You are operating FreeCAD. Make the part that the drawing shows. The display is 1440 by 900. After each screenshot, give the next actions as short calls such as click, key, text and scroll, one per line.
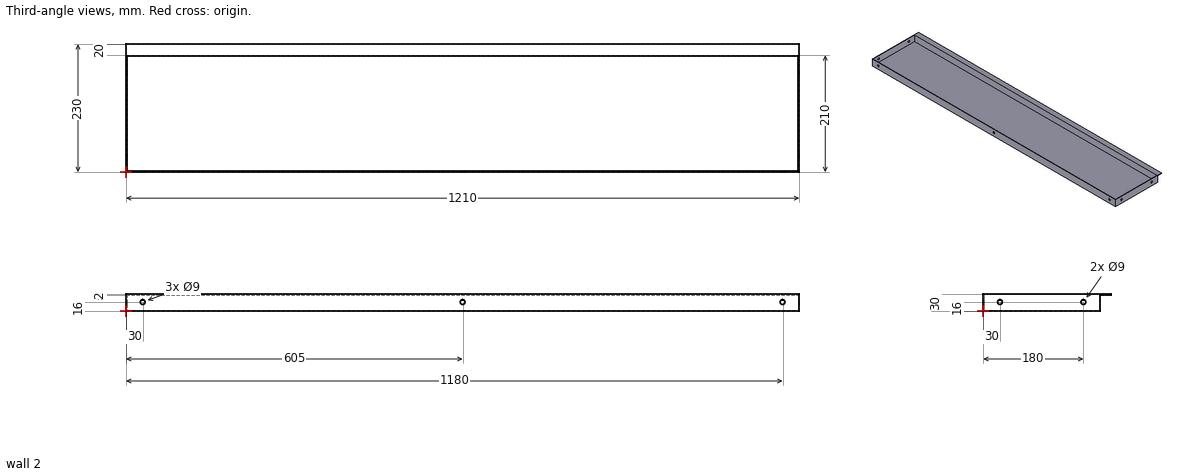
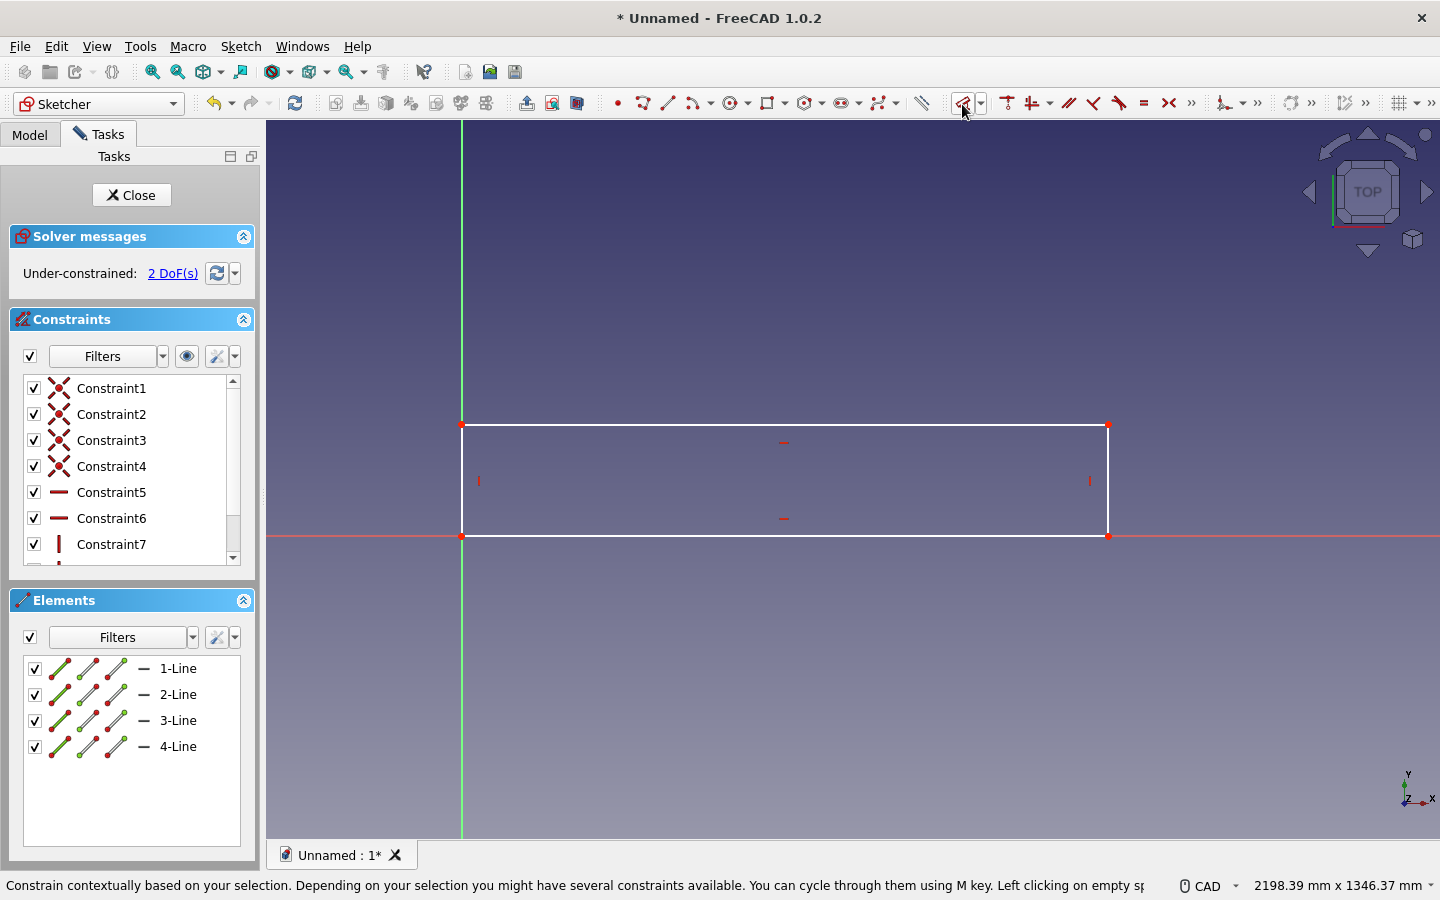
click(1108, 503)
click(1142, 481)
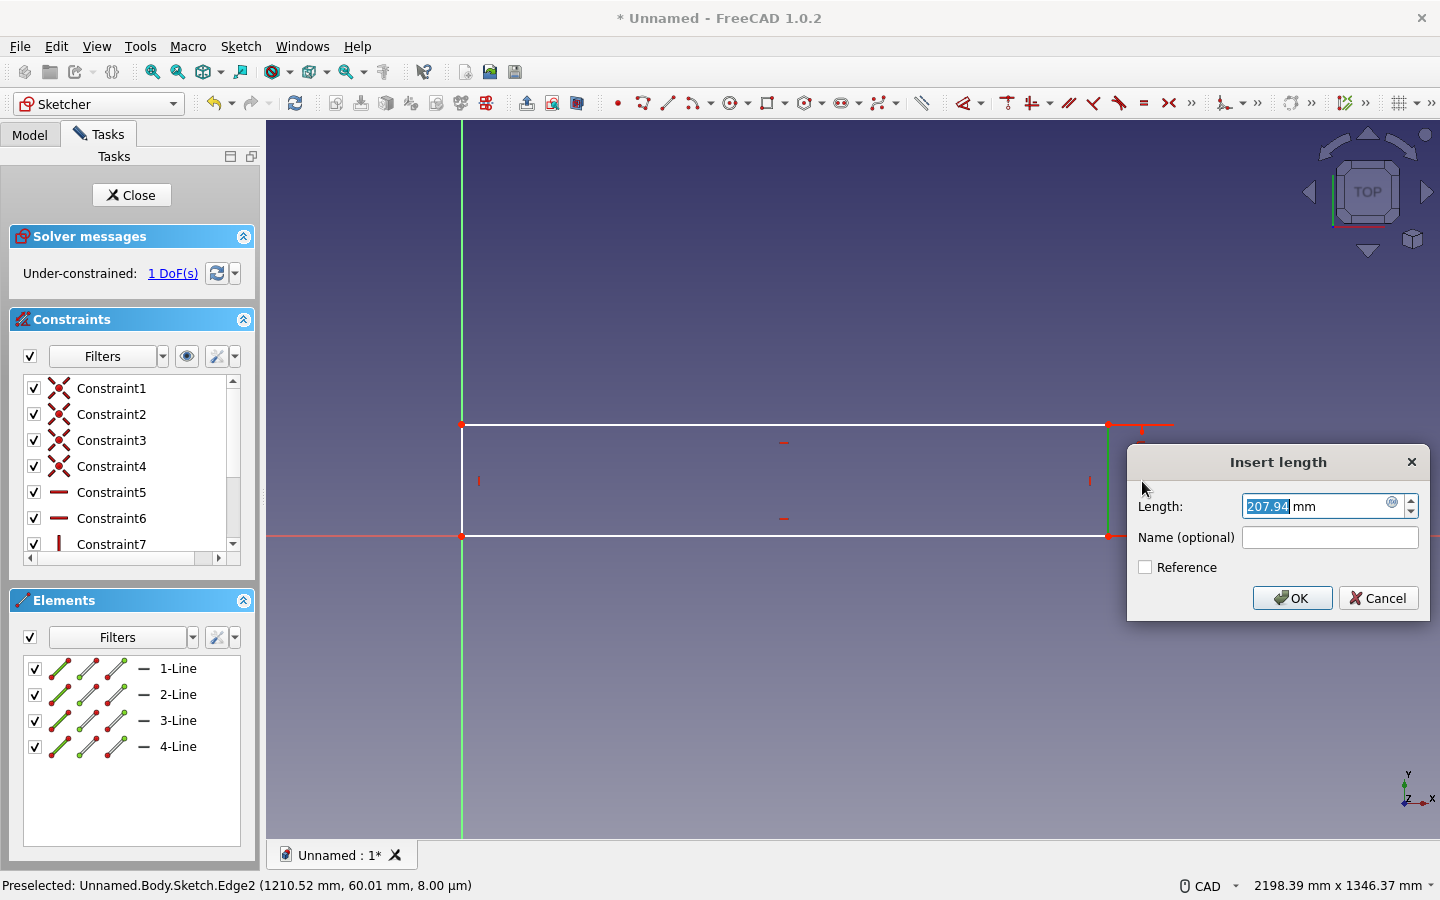
text(210)
key(Return)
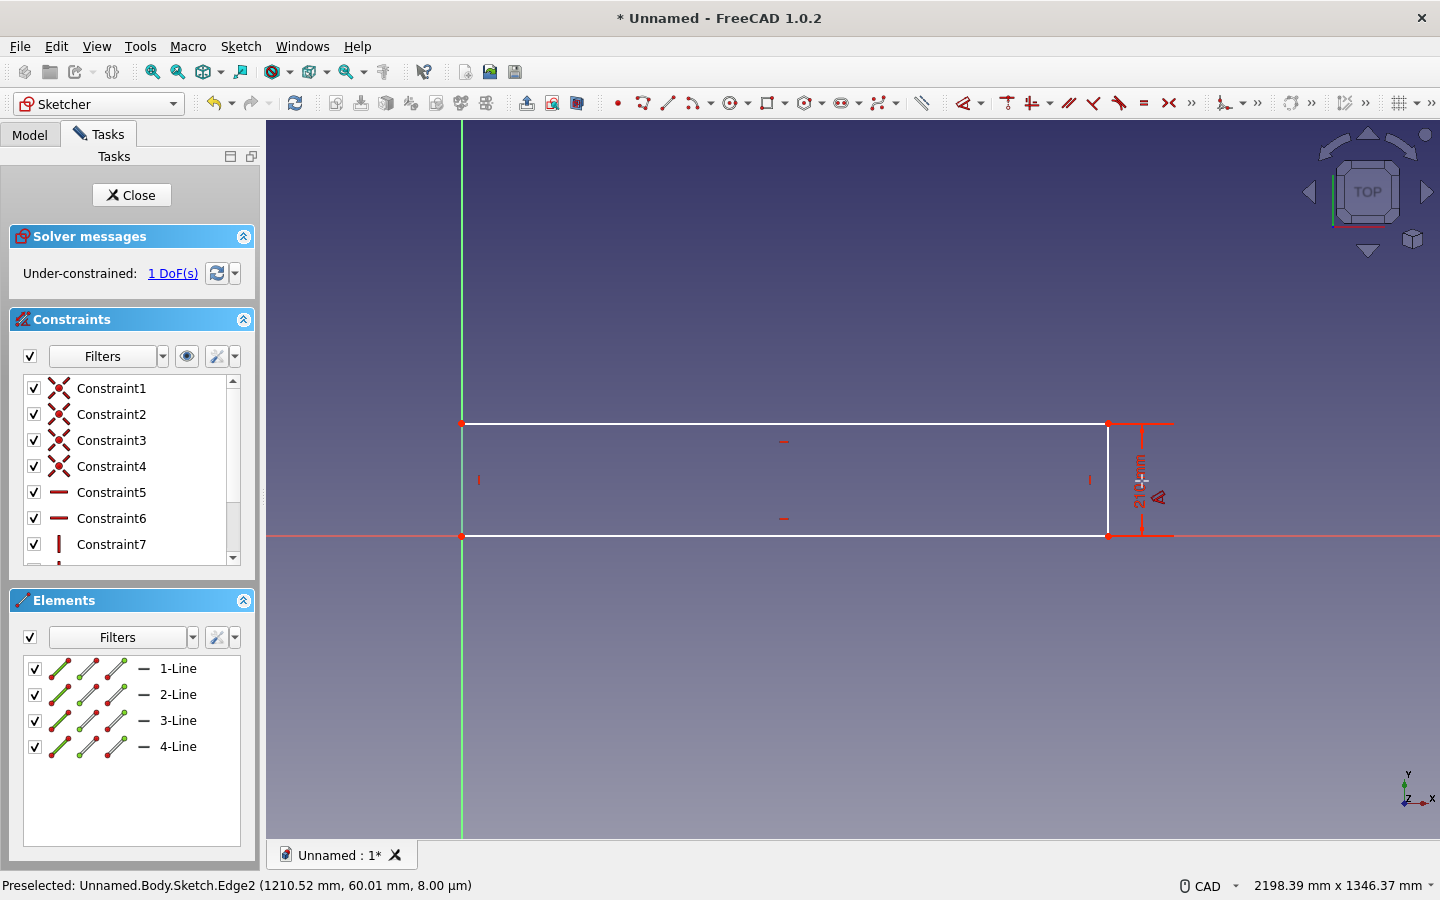
click(655, 536)
click(785, 570)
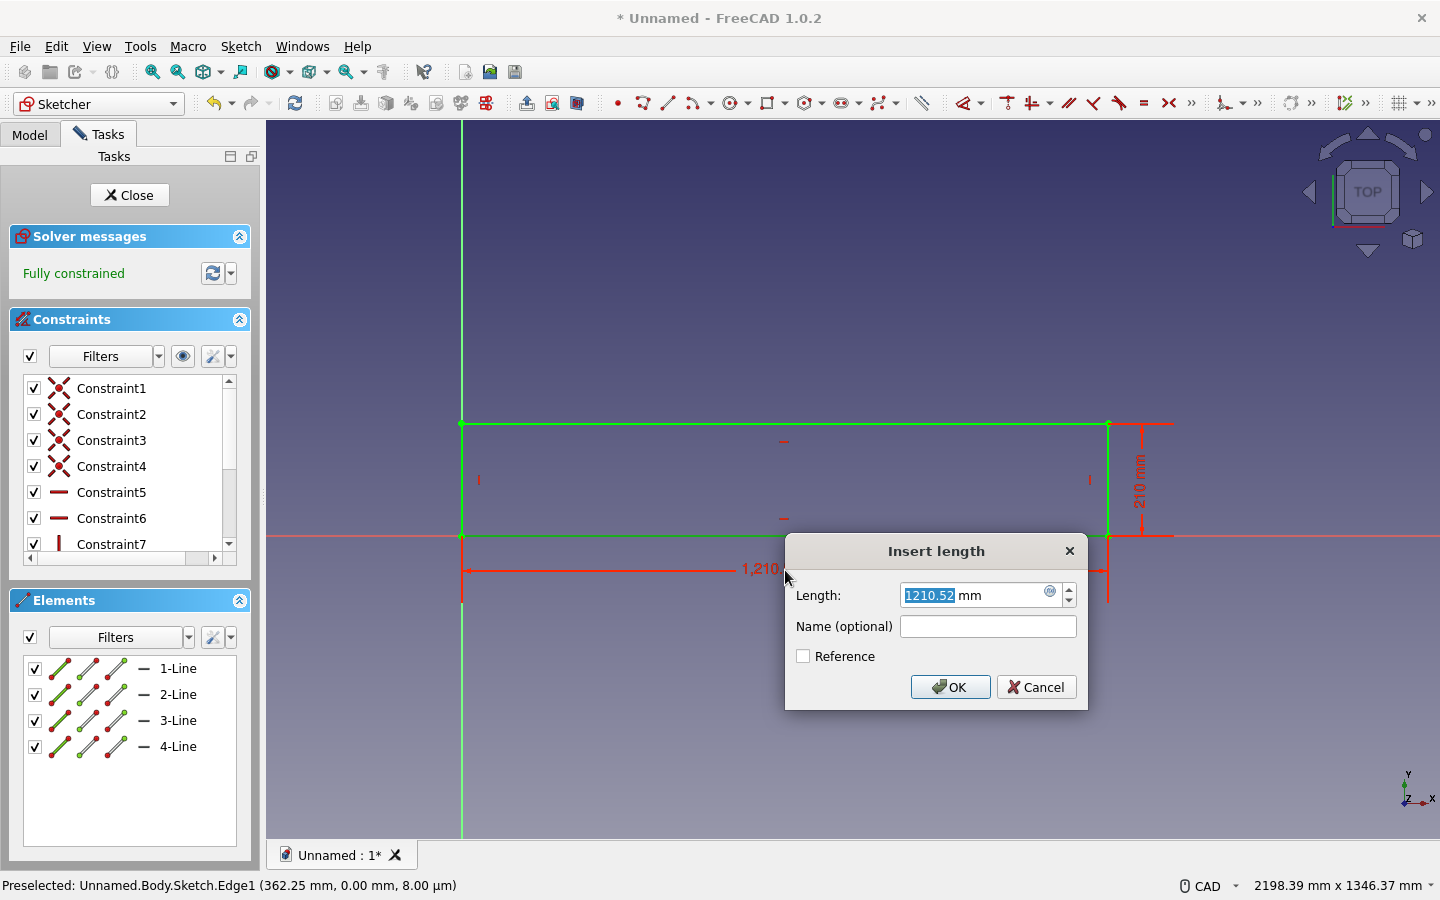
text(1210)
key(Return)
key(Escape)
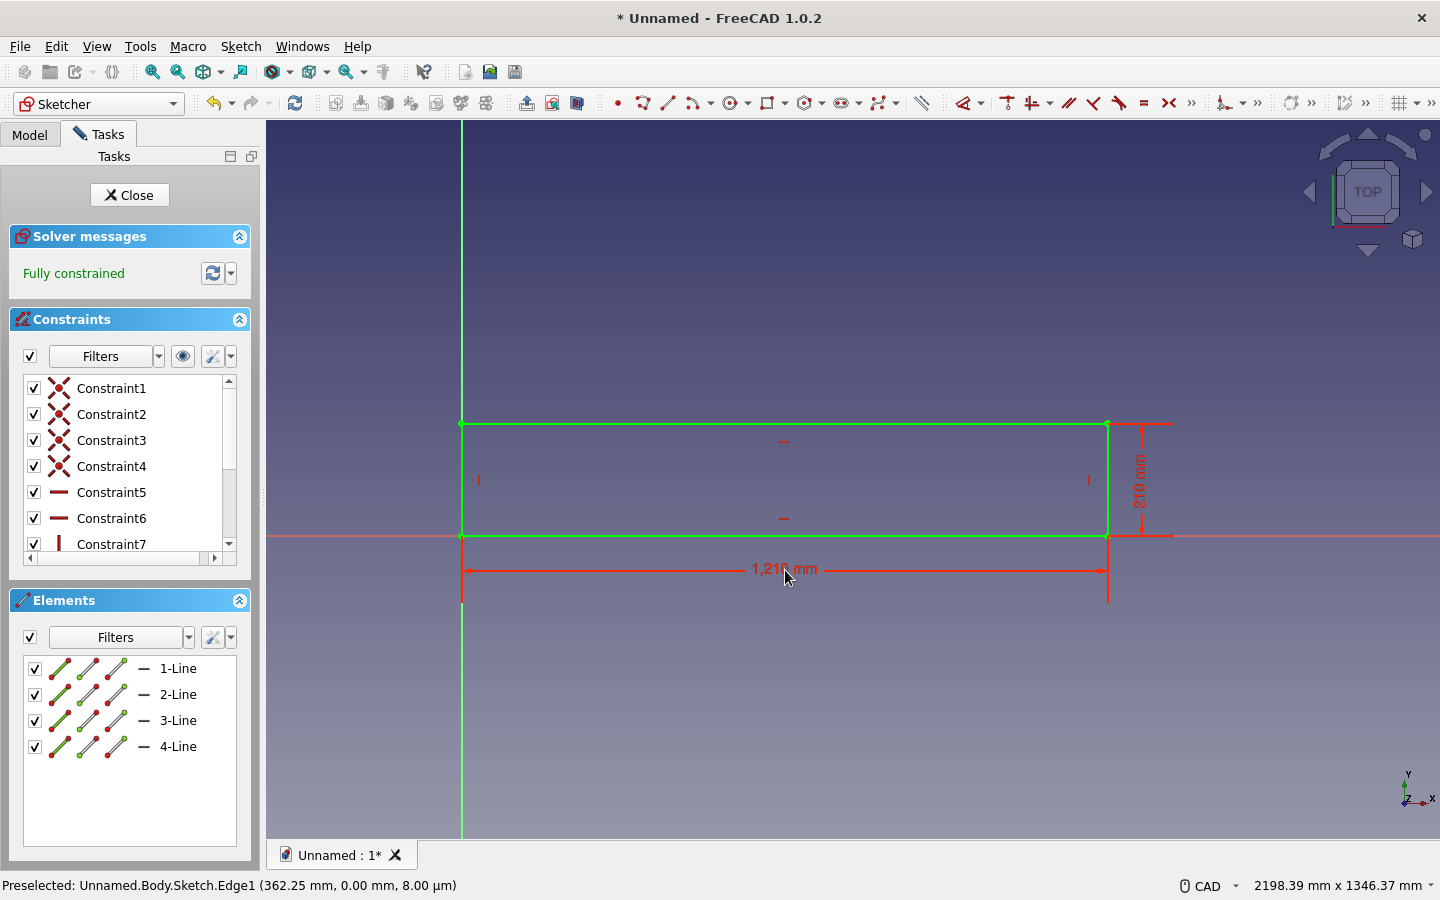
click(130, 195)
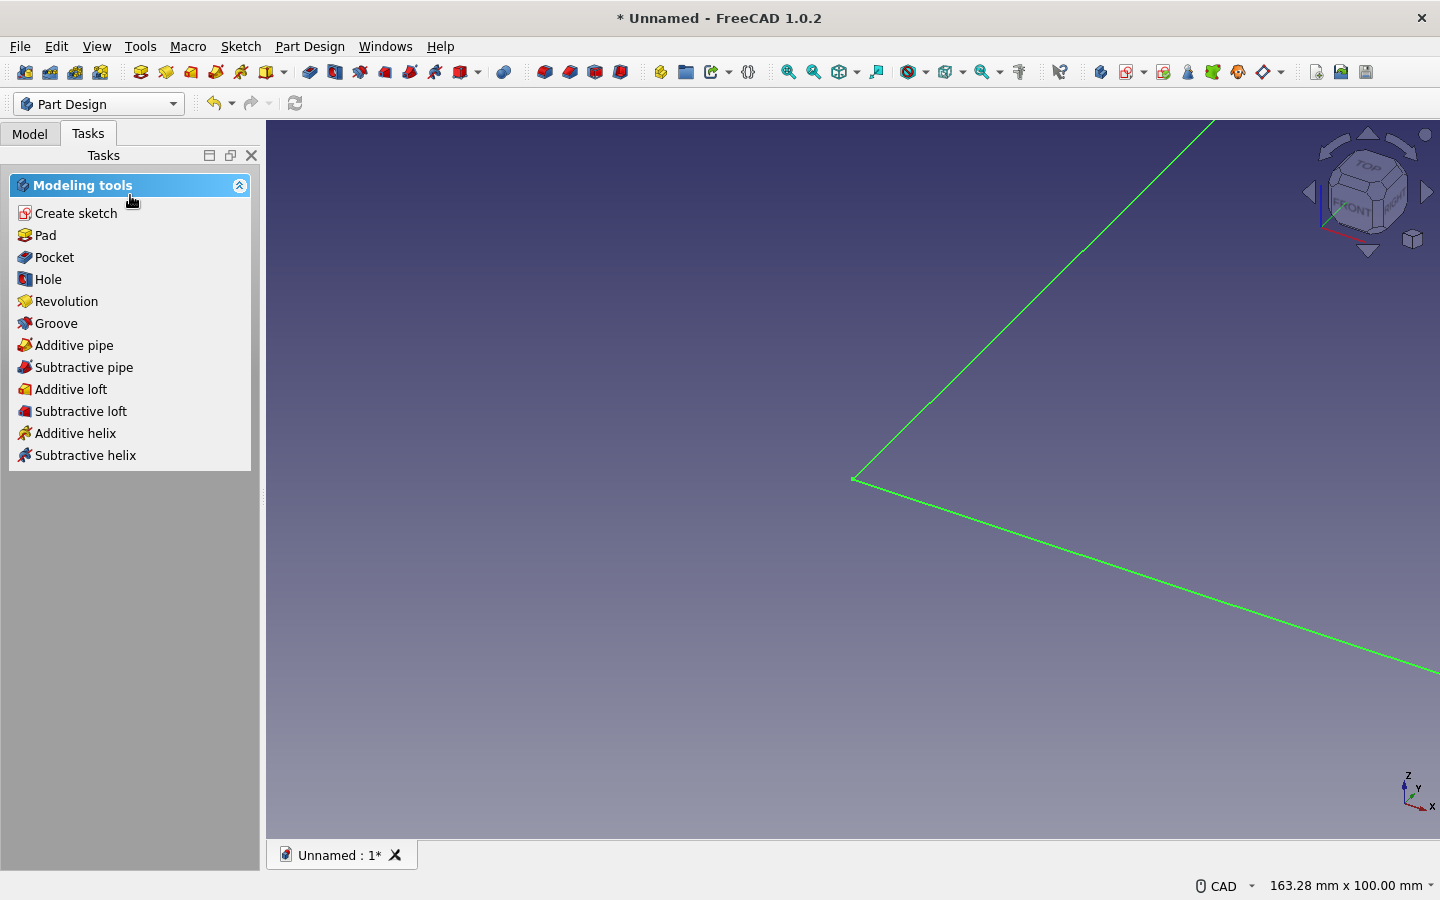
click(141, 72)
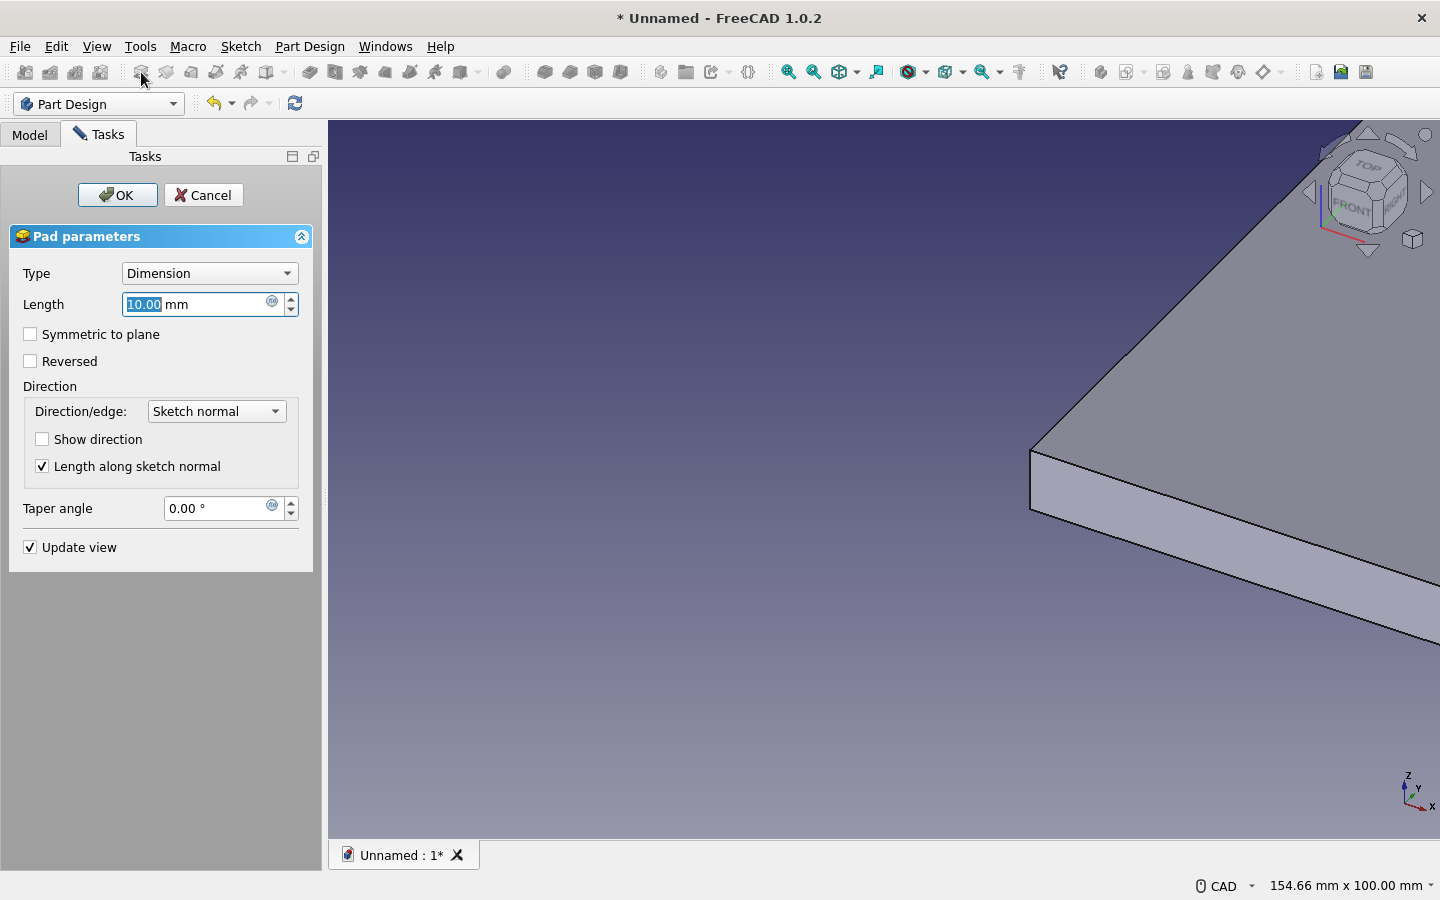
text(30)
key(Tab)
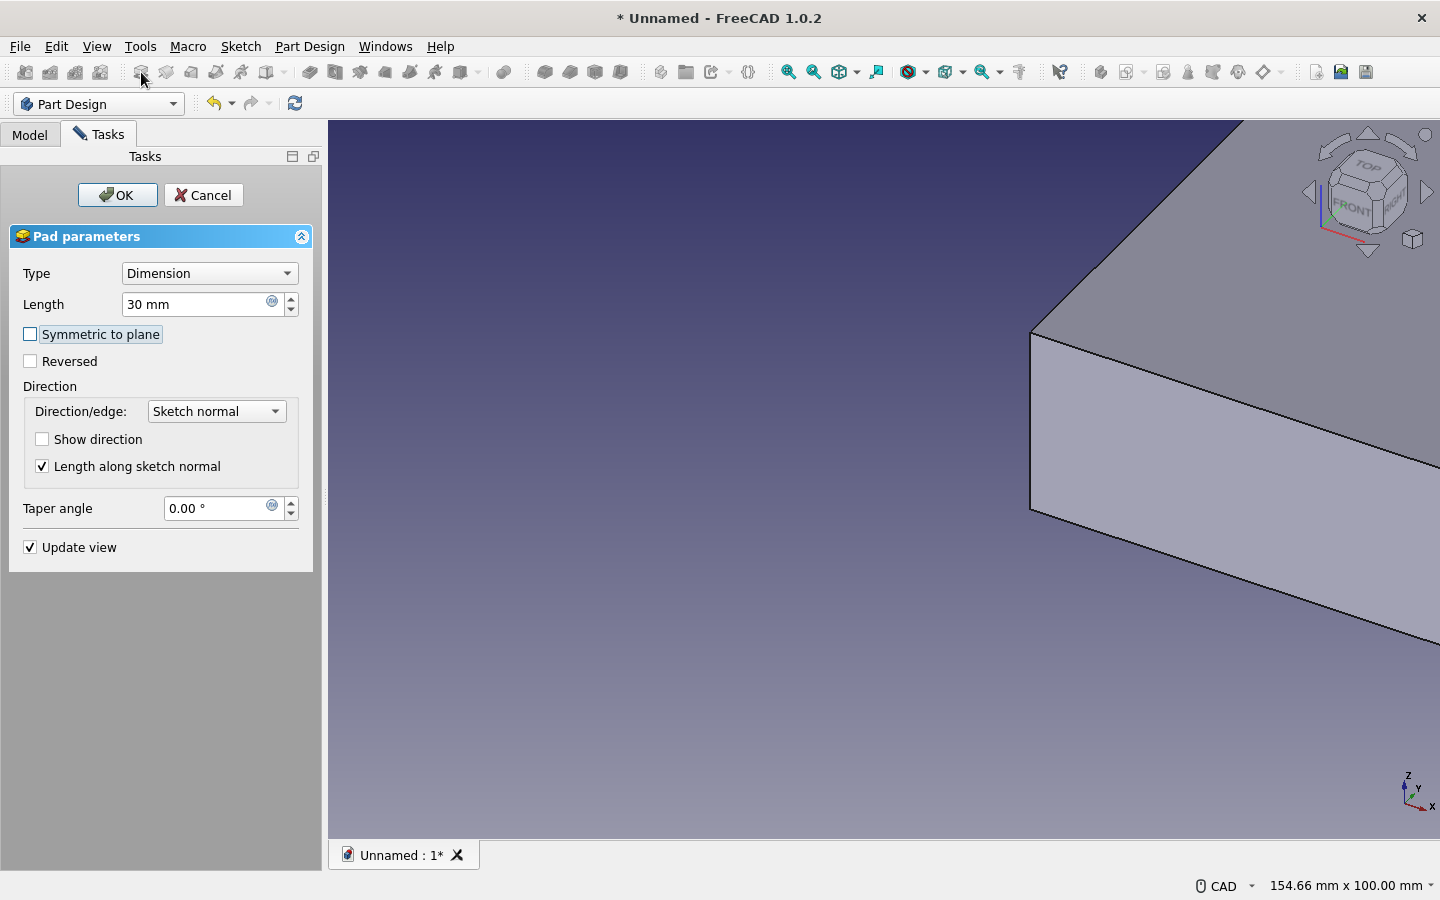
click(118, 195)